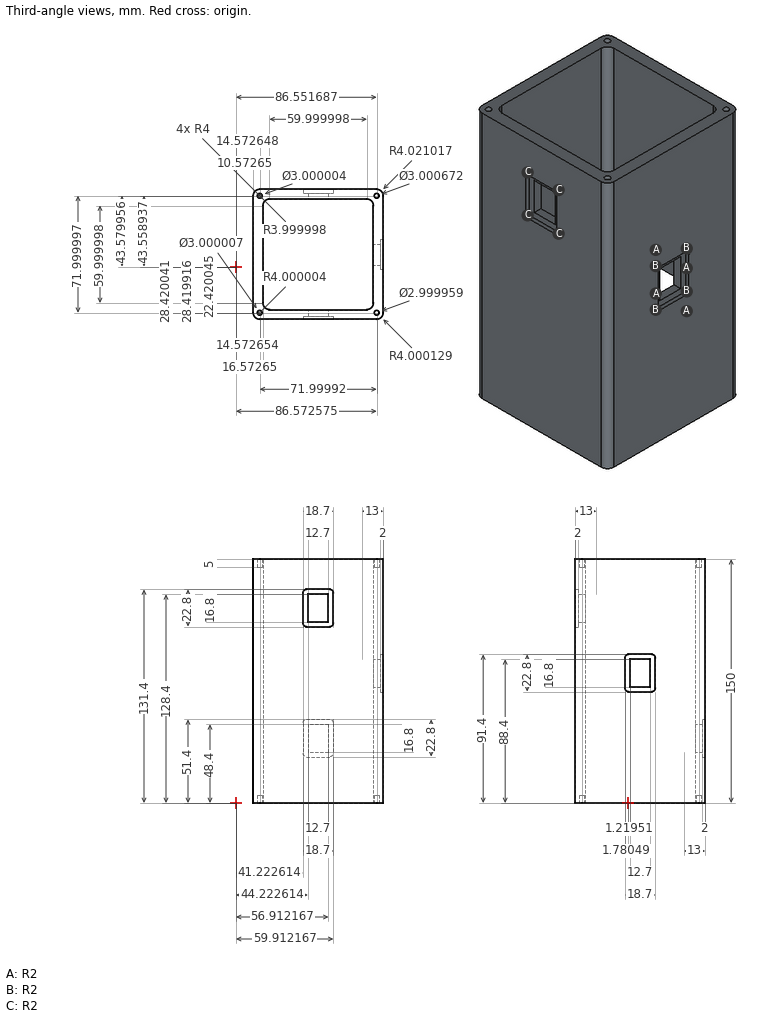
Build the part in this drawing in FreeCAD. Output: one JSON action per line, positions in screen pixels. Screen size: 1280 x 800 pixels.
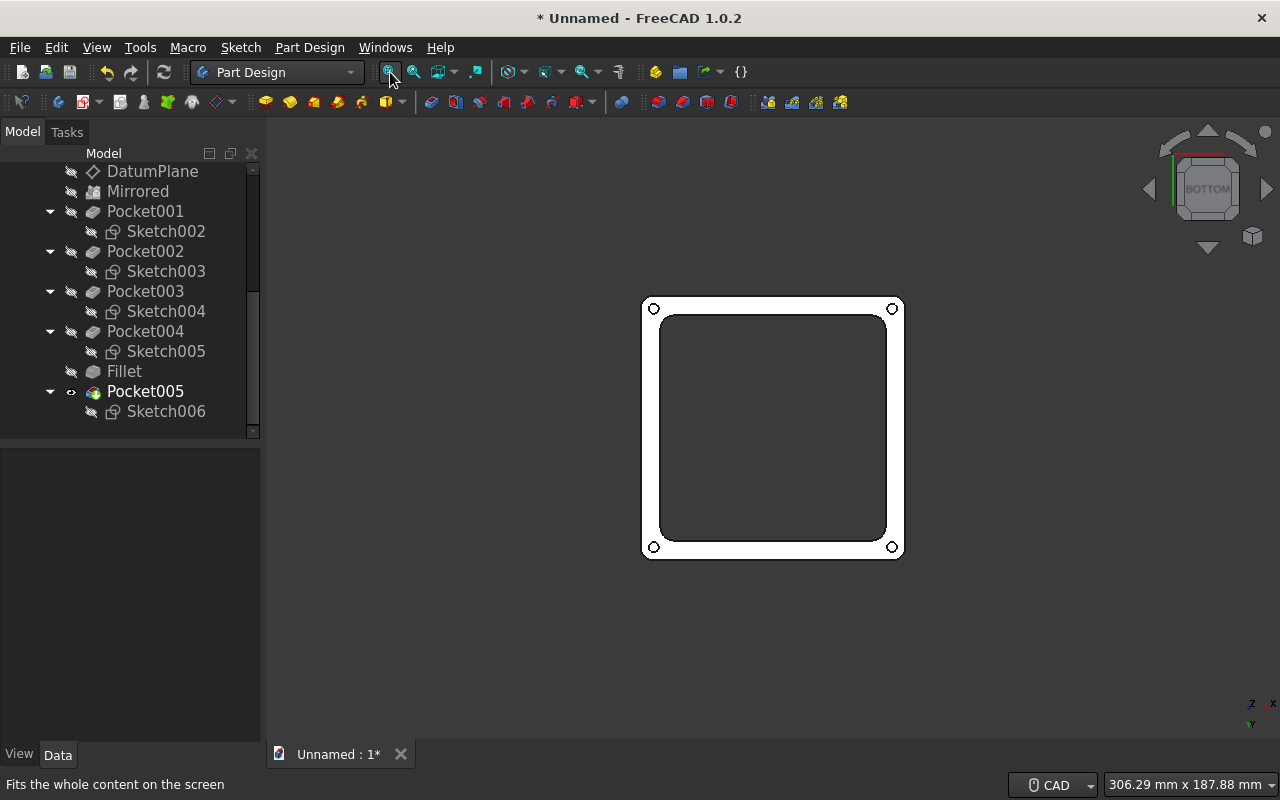
{"action": "scroll", "coordinate": [902, 458], "scroll_direction": "up", "scroll_amount": 9}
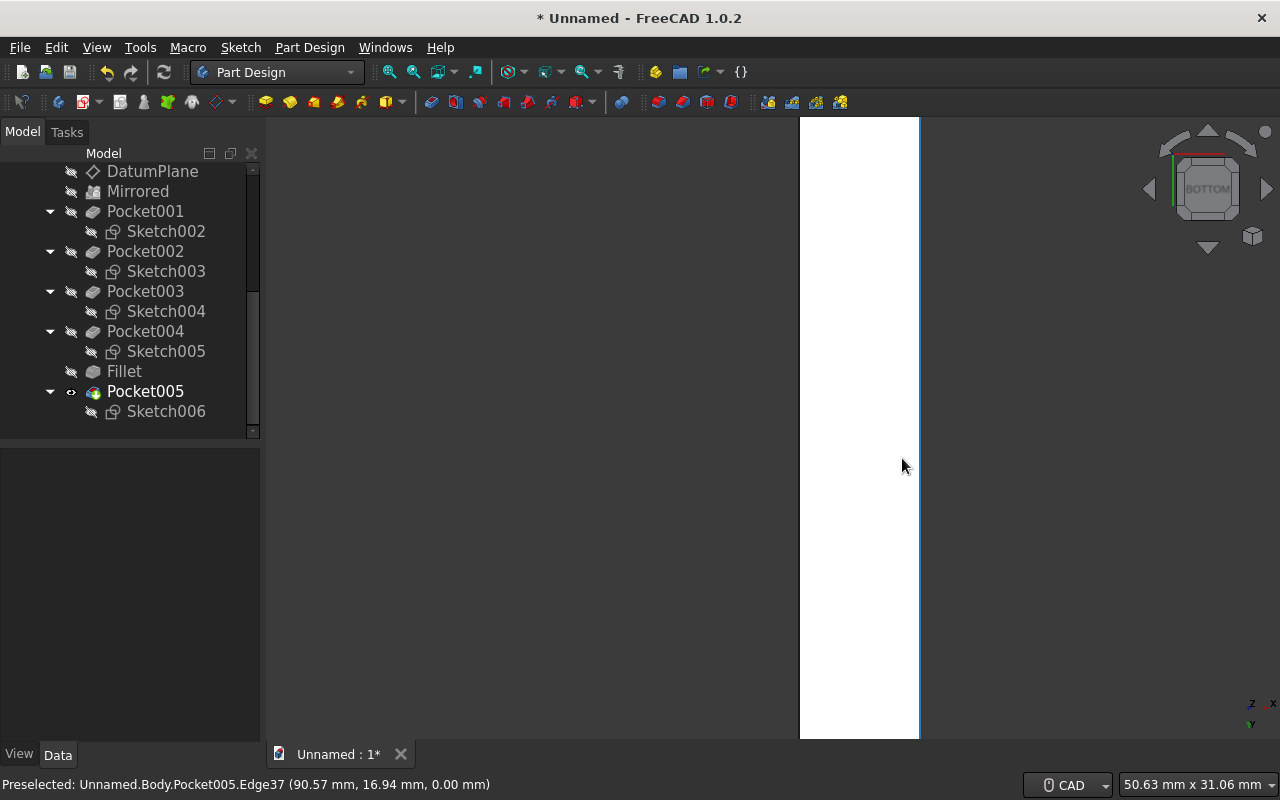
{"action": "left_click", "coordinate": [390, 72]}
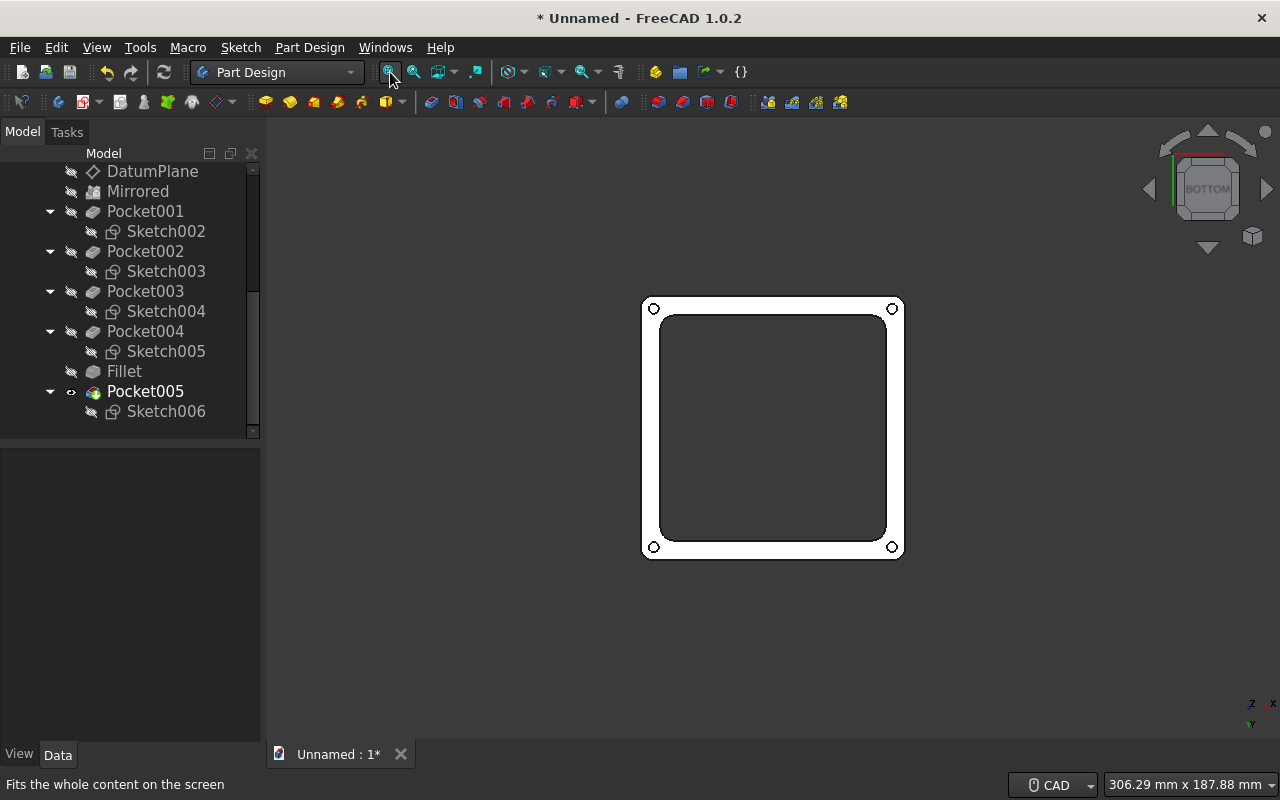
{"action": "key", "text": "4"}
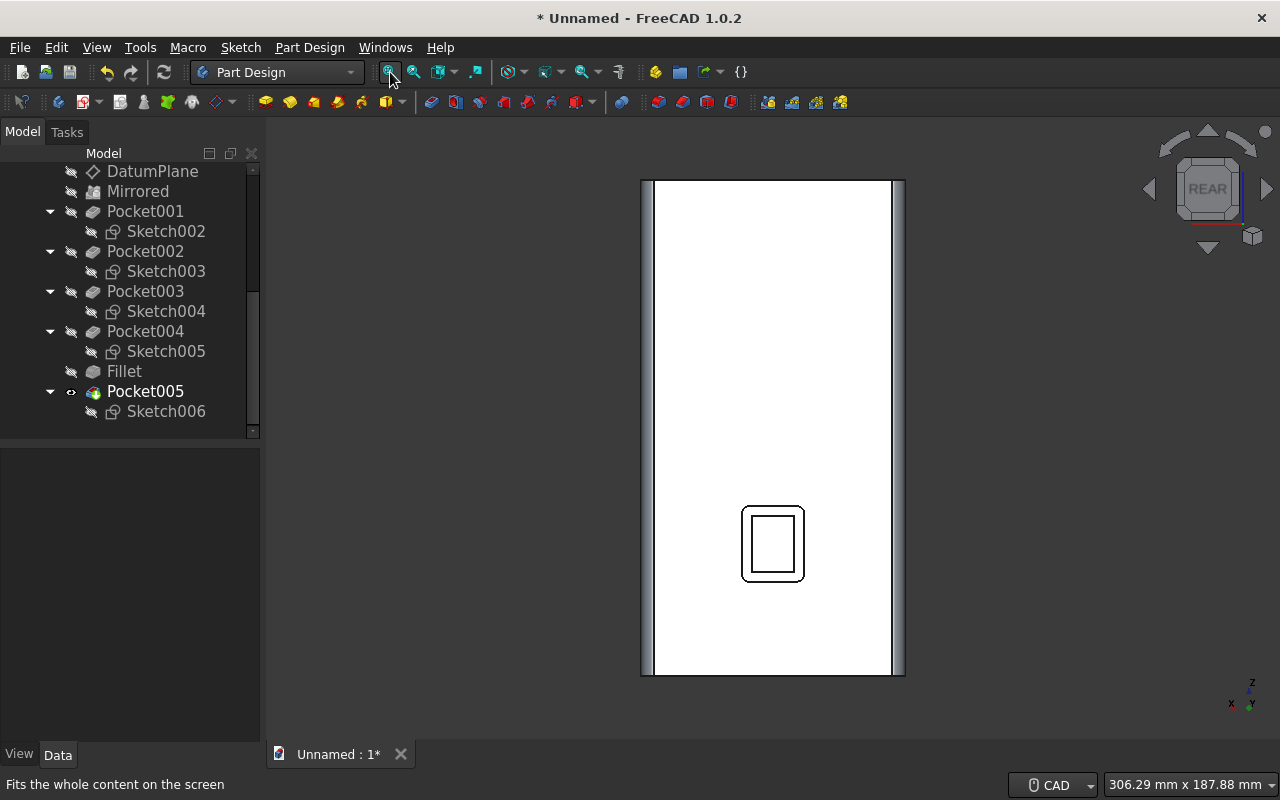
{"action": "scroll", "coordinate": [644, 373], "scroll_direction": "up", "scroll_amount": 9}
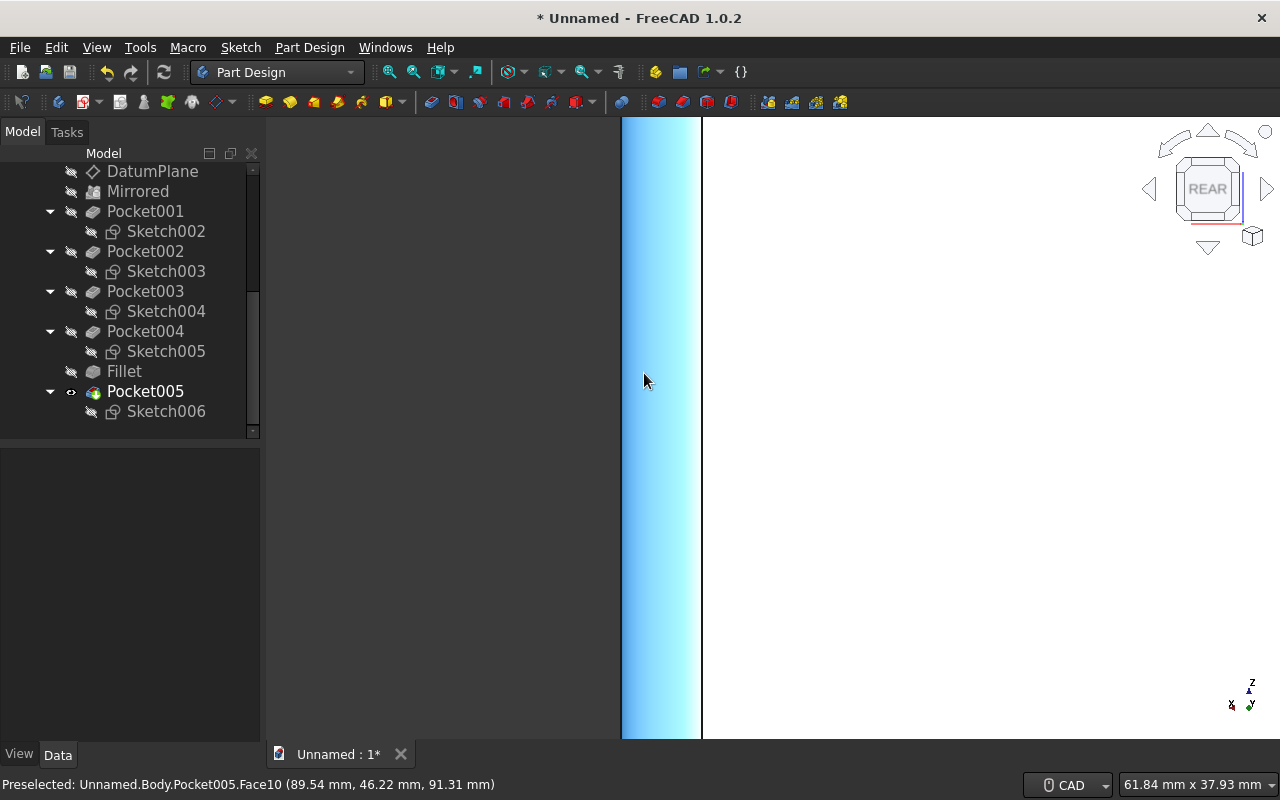
{"action": "left_click", "coordinate": [390, 72]}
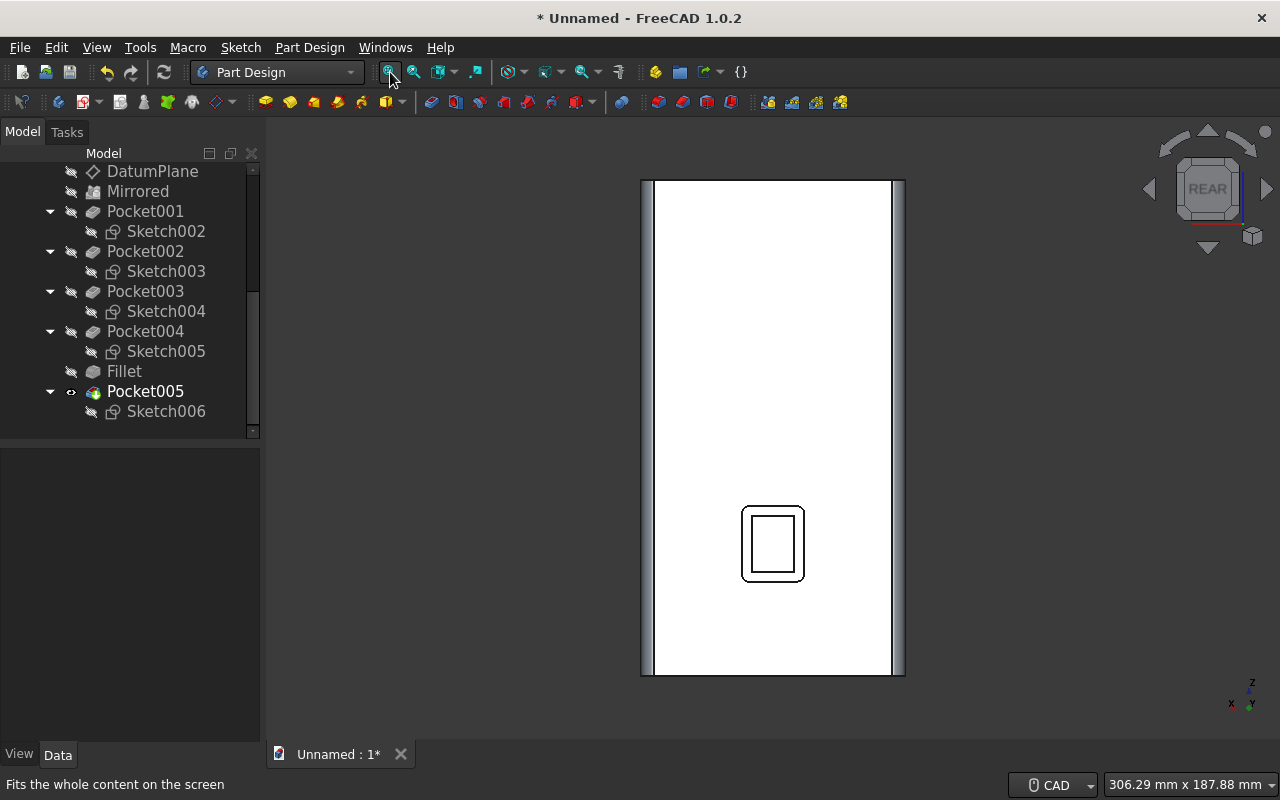
{"action": "key", "text": "6"}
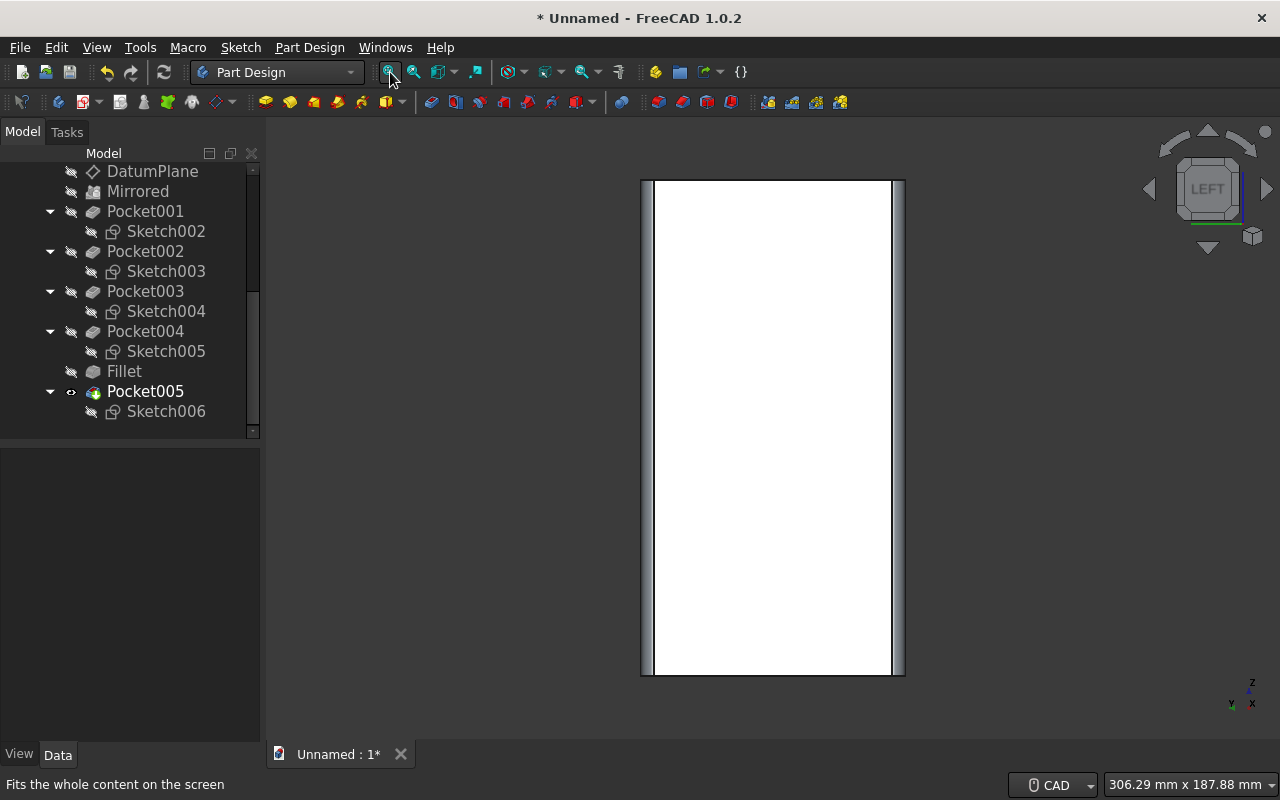
{"action": "scroll", "coordinate": [742, 373], "scroll_direction": "up", "scroll_amount": 9}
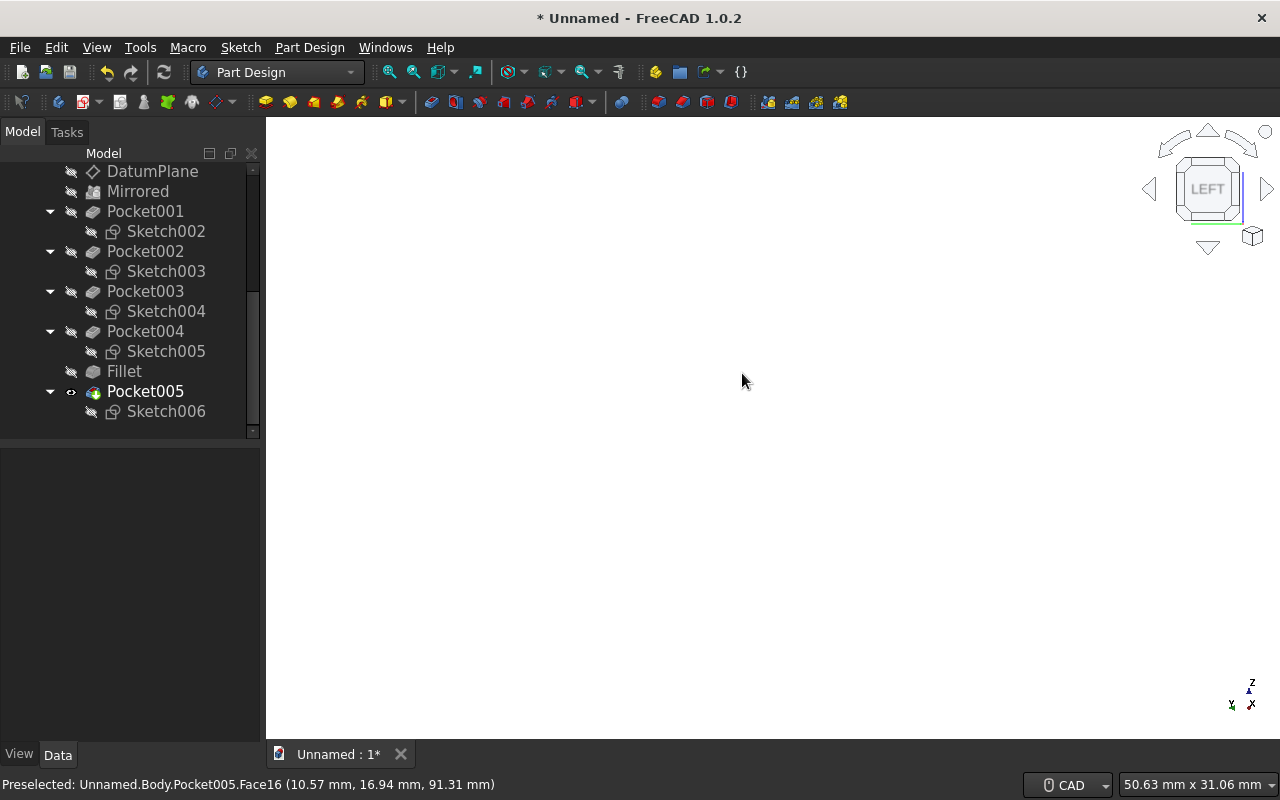
{"action": "left_click", "coordinate": [390, 72]}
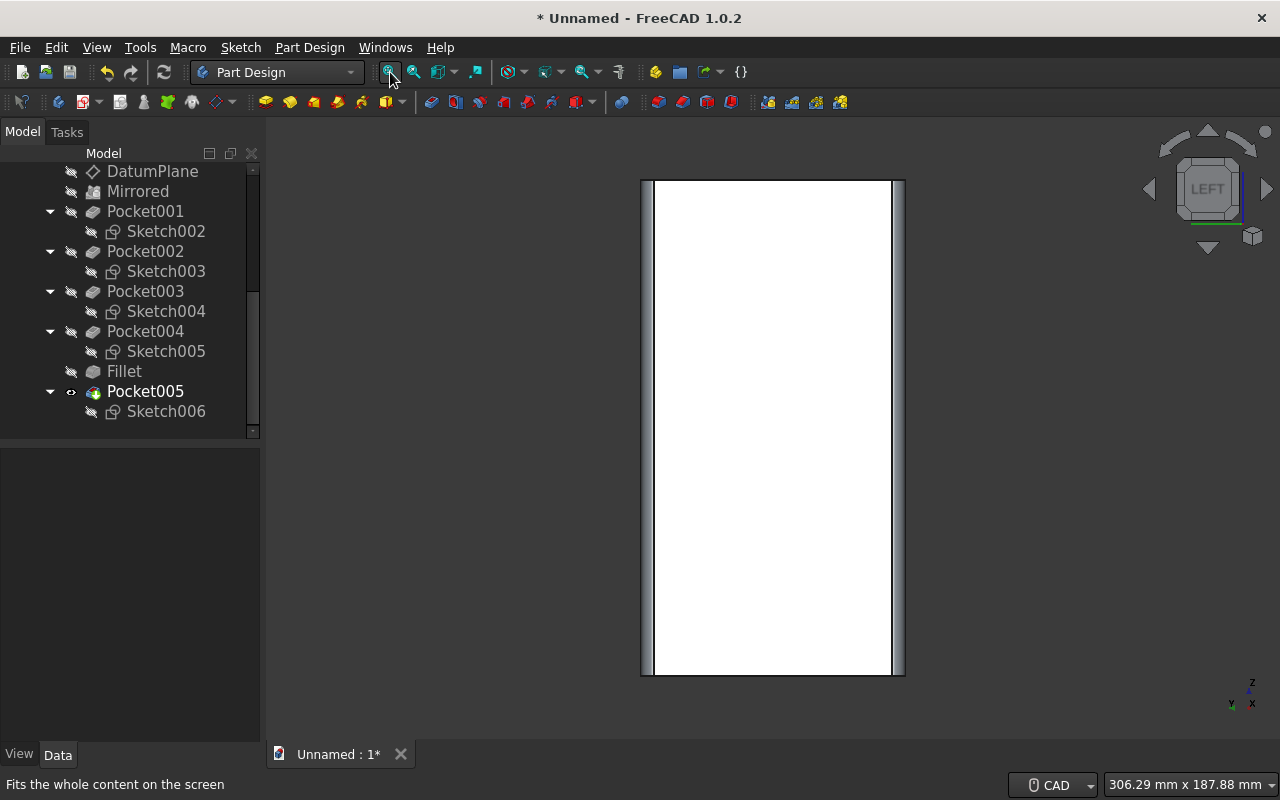
{"action": "key", "text": "v 3"}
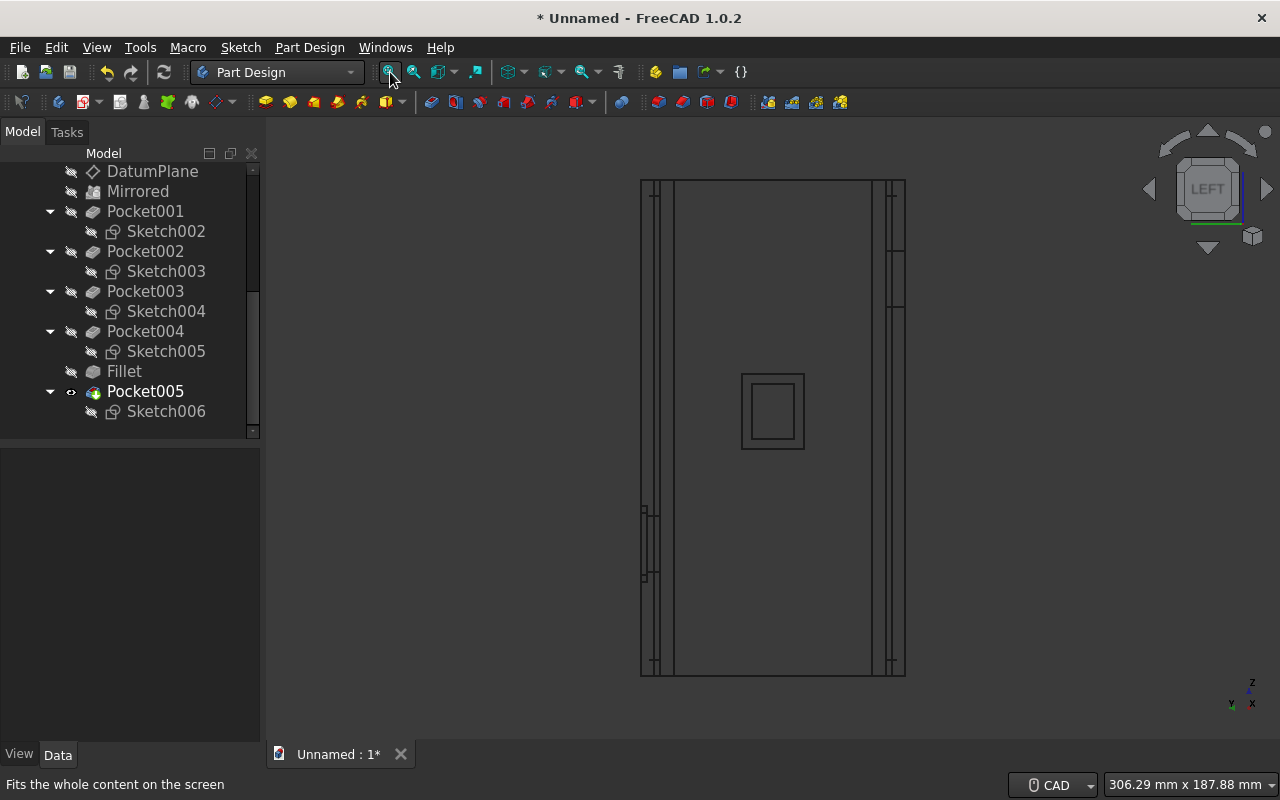
{"action": "key", "text": "0"}